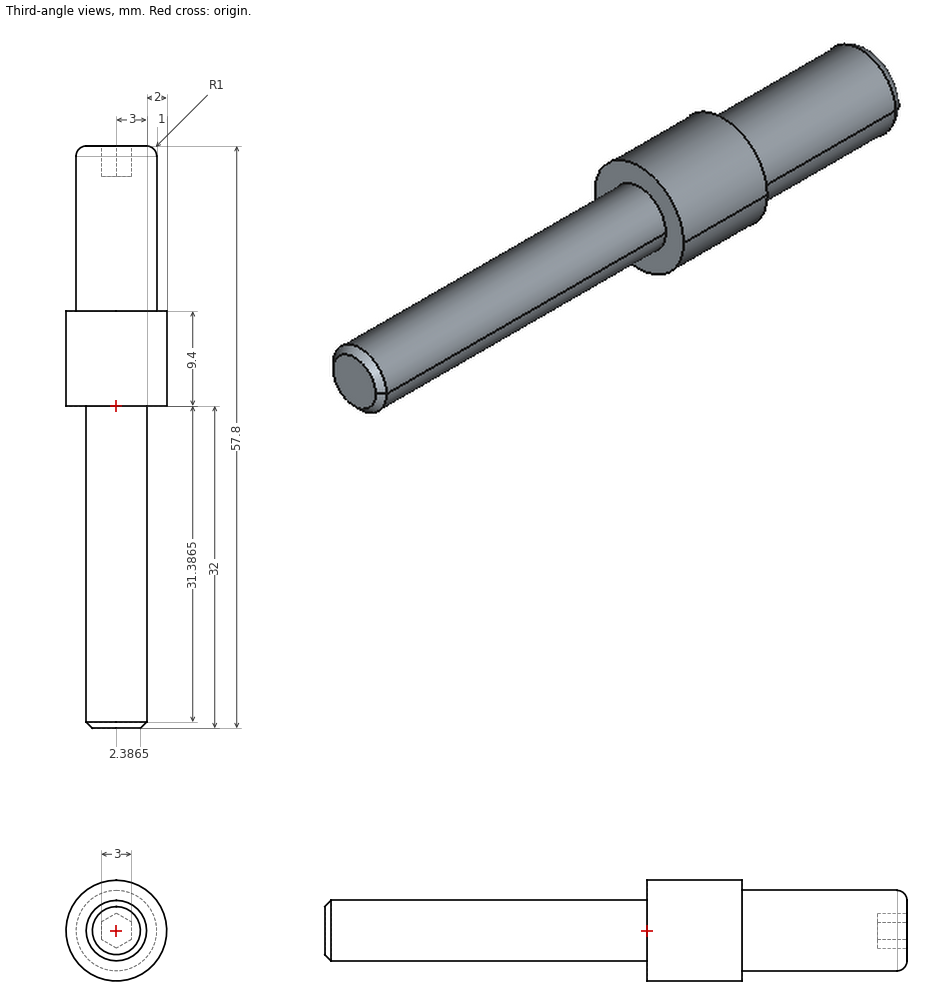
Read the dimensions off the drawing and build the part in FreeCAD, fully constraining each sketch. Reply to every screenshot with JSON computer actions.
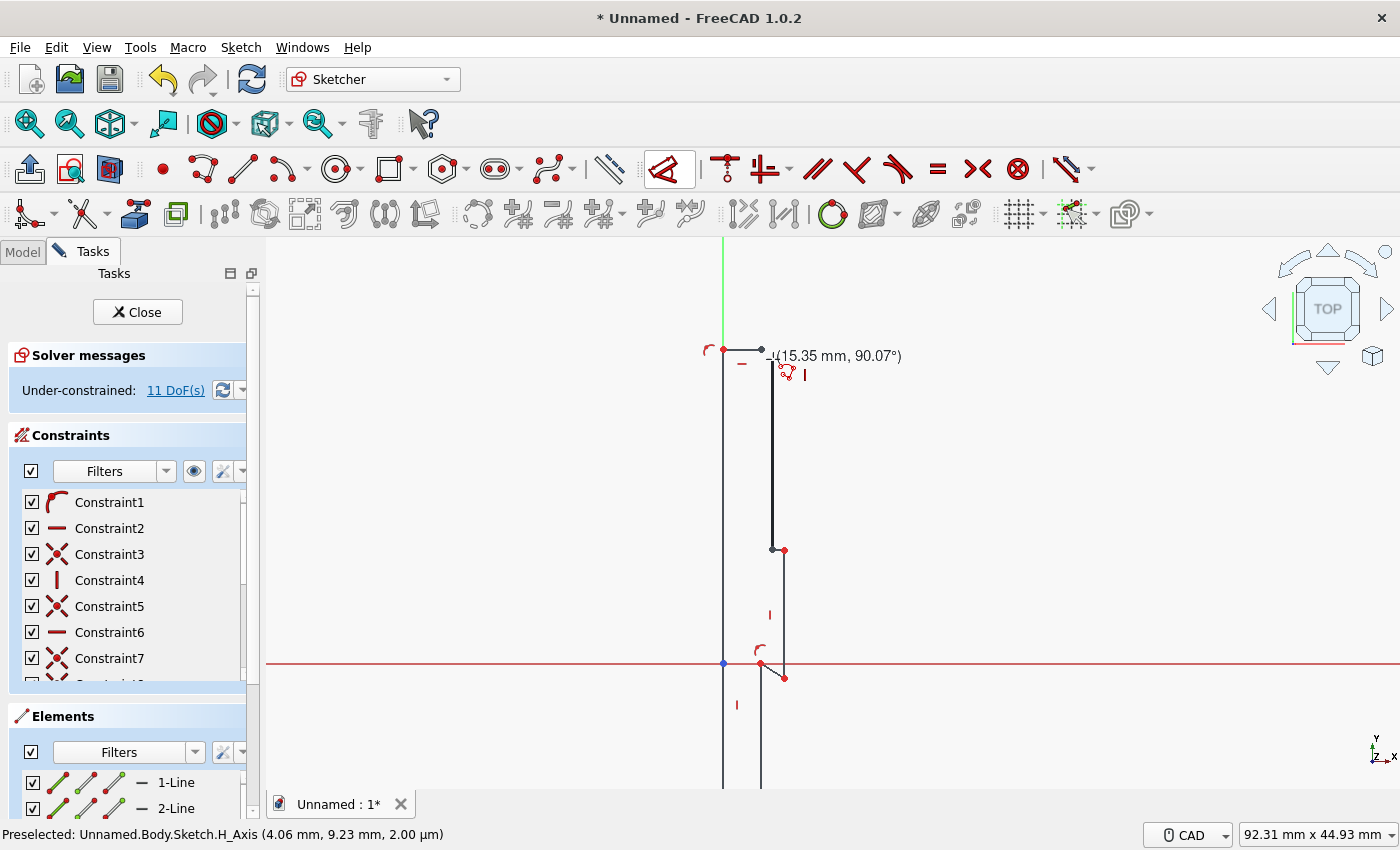
{"action": "left_click", "coordinate": [773, 359]}
{"action": "right_click", "coordinate": [773, 359]}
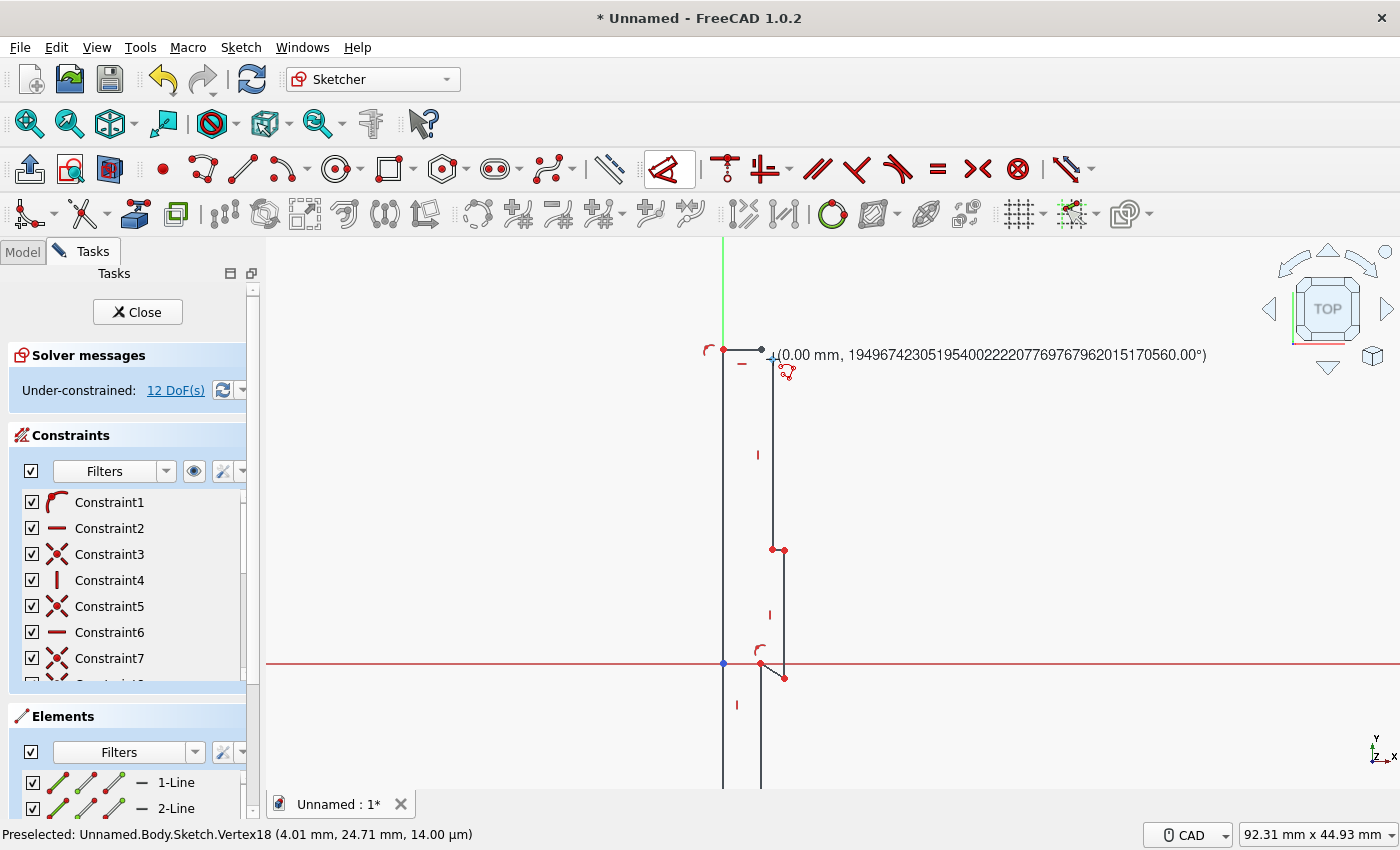
{"action": "left_click", "coordinate": [310, 170]}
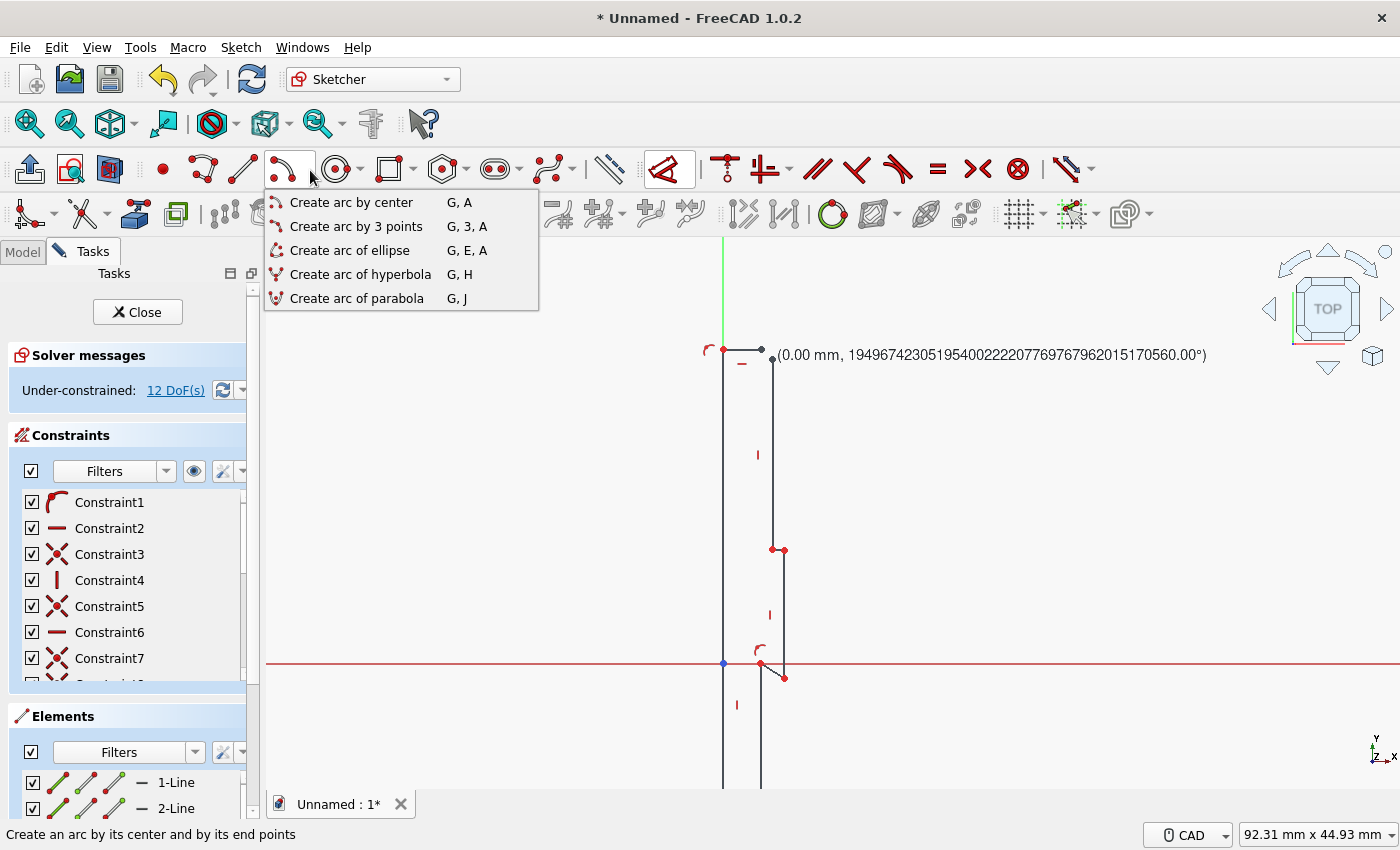
{"action": "left_click", "coordinate": [402, 226]}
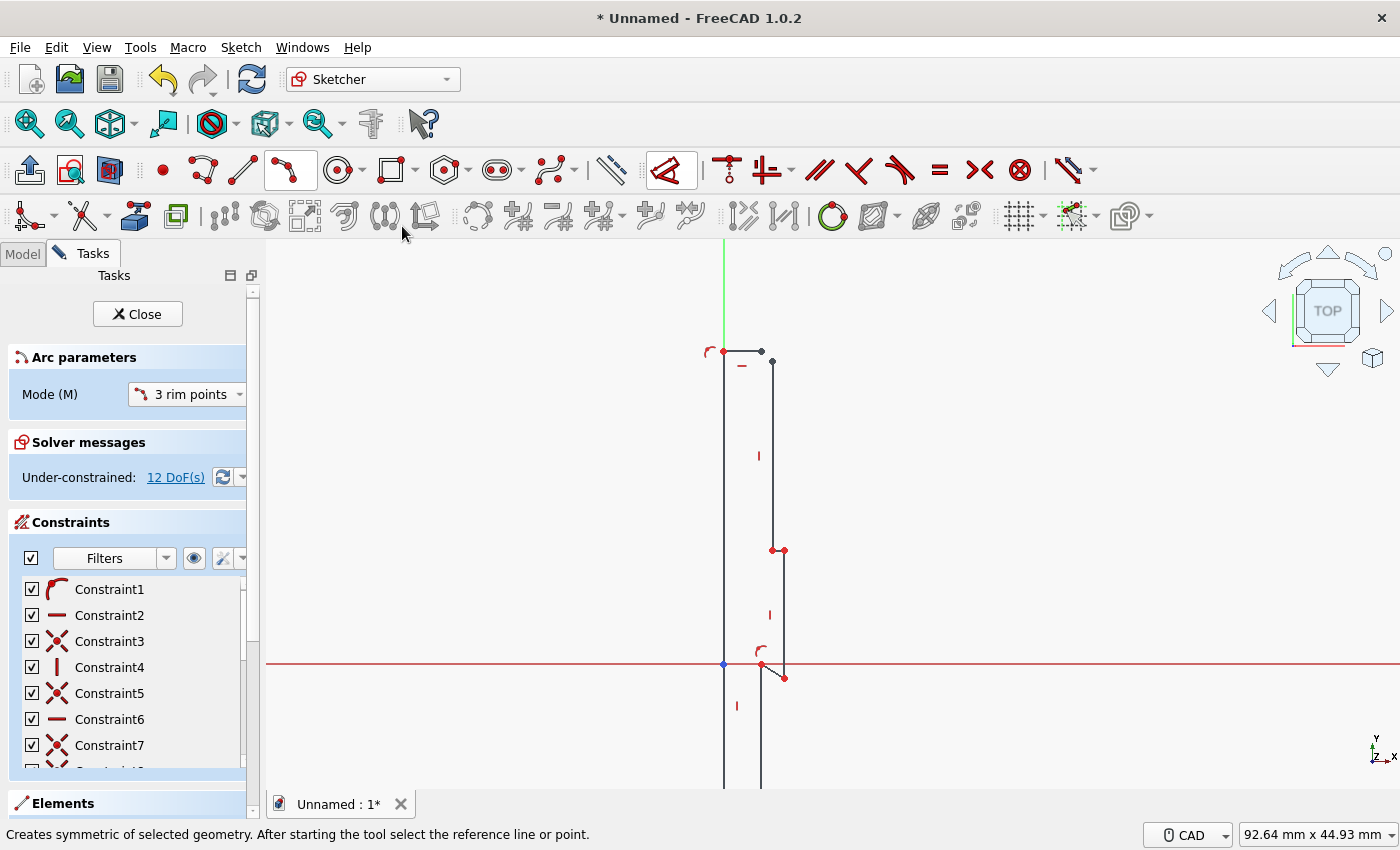
{"action": "left_click", "coordinate": [773, 362]}
{"action": "left_click", "coordinate": [762, 351]}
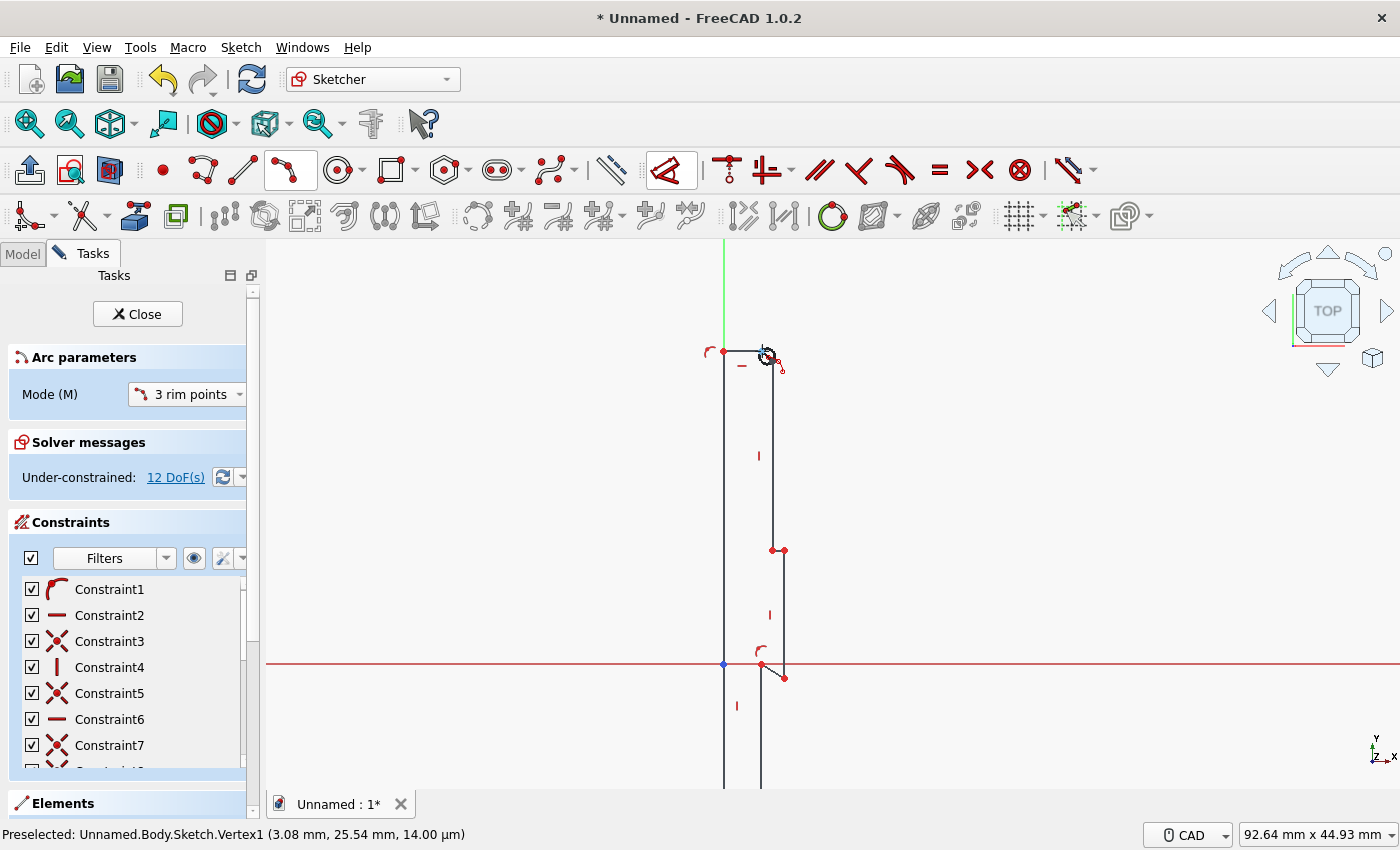
{"action": "scroll", "coordinate": [769, 352], "scroll_direction": "up", "scroll_amount": 8}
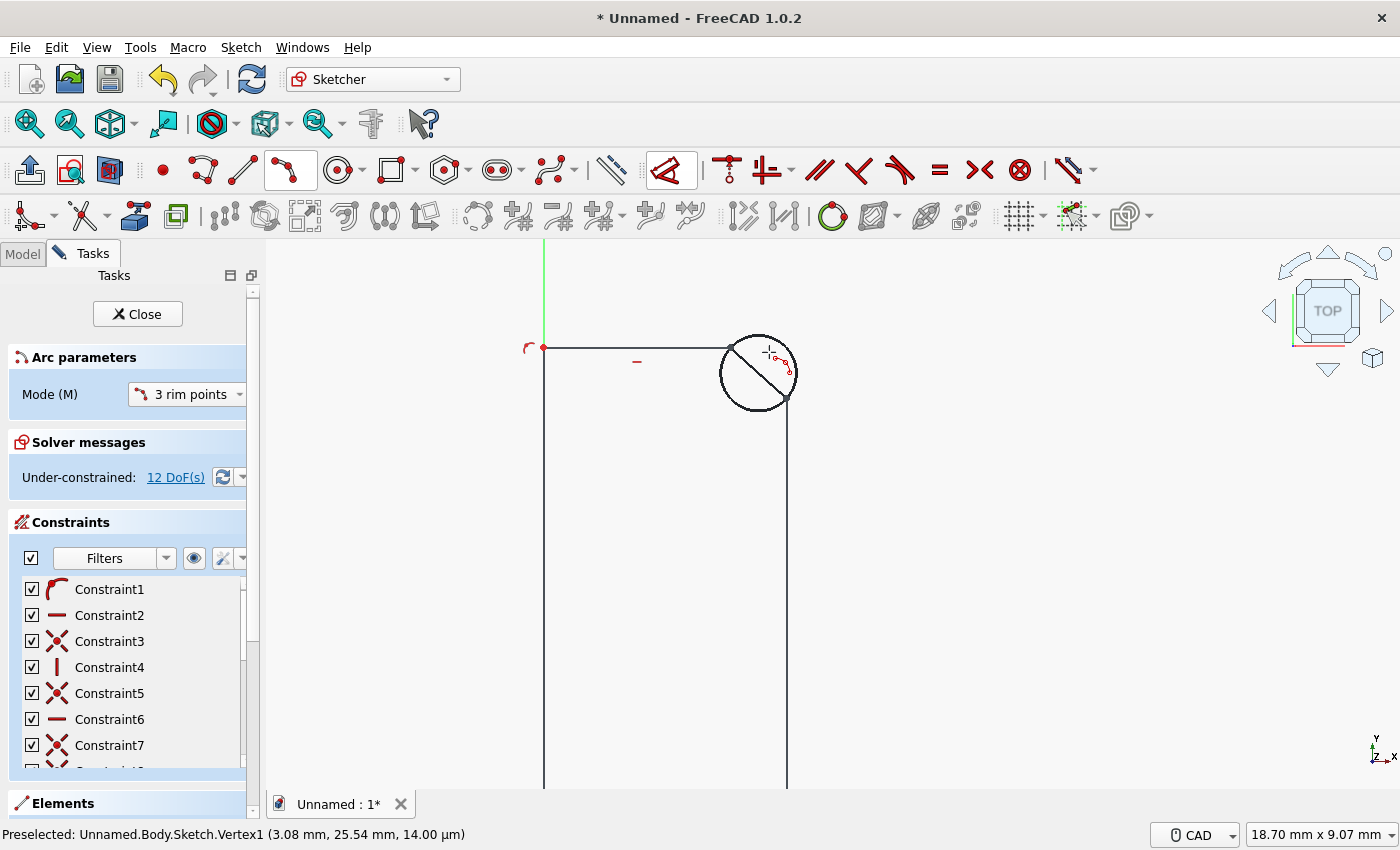
{"action": "left_click", "coordinate": [768, 350]}
{"action": "key", "text": "Escape"}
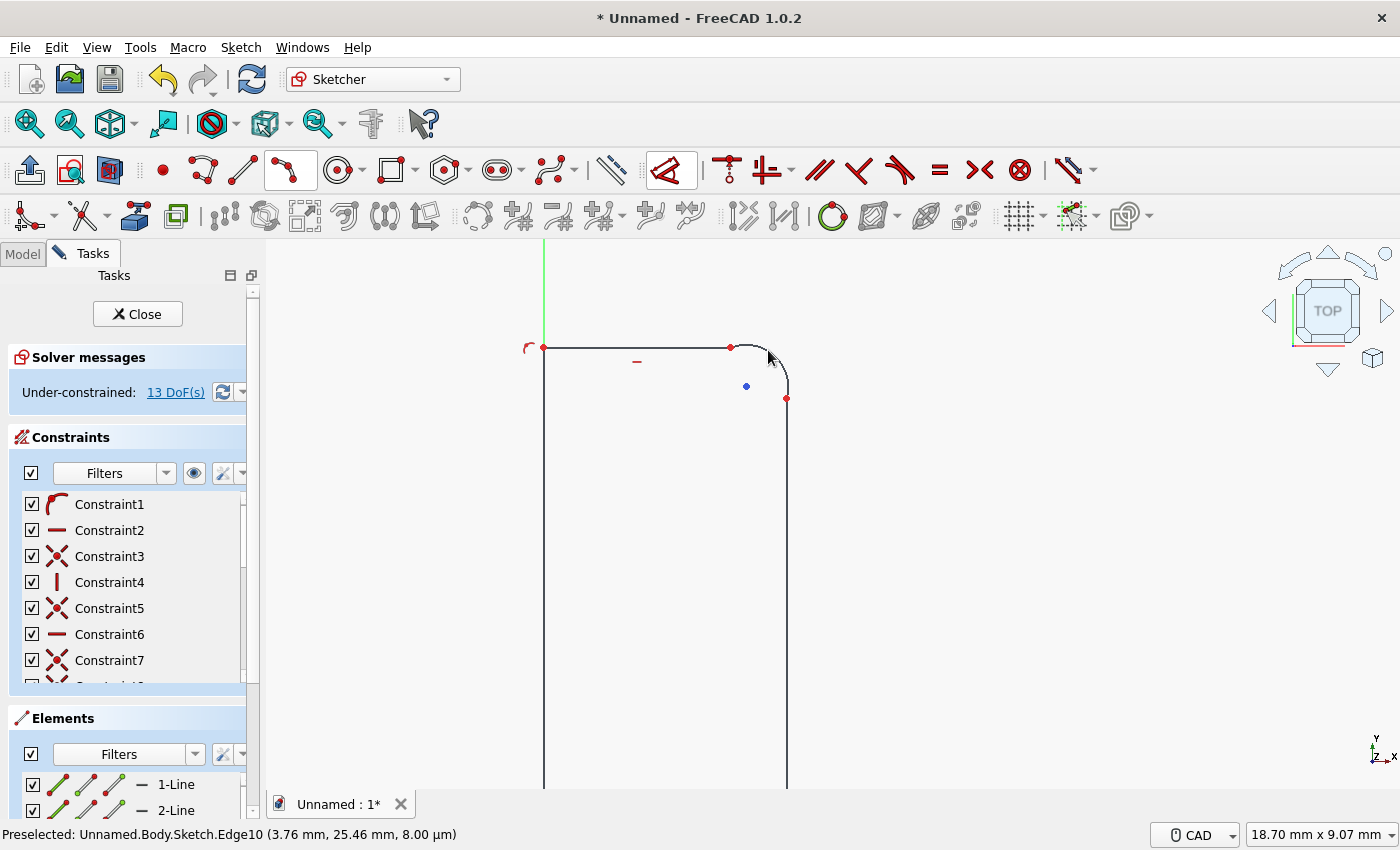
{"action": "scroll", "coordinate": [771, 357], "scroll_direction": "down", "scroll_amount": 12}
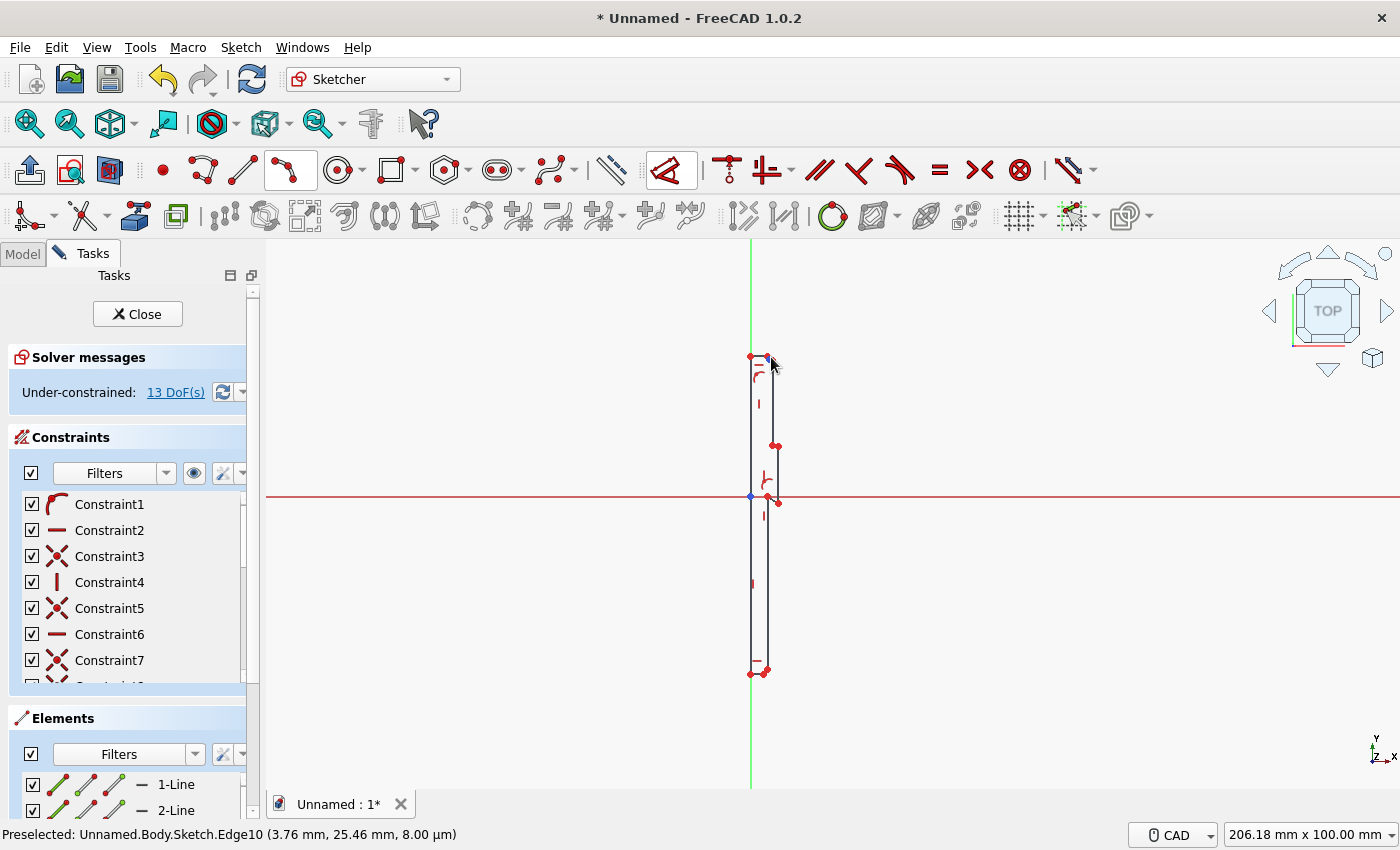
{"action": "scroll", "coordinate": [763, 356], "scroll_direction": "up", "scroll_amount": 5}